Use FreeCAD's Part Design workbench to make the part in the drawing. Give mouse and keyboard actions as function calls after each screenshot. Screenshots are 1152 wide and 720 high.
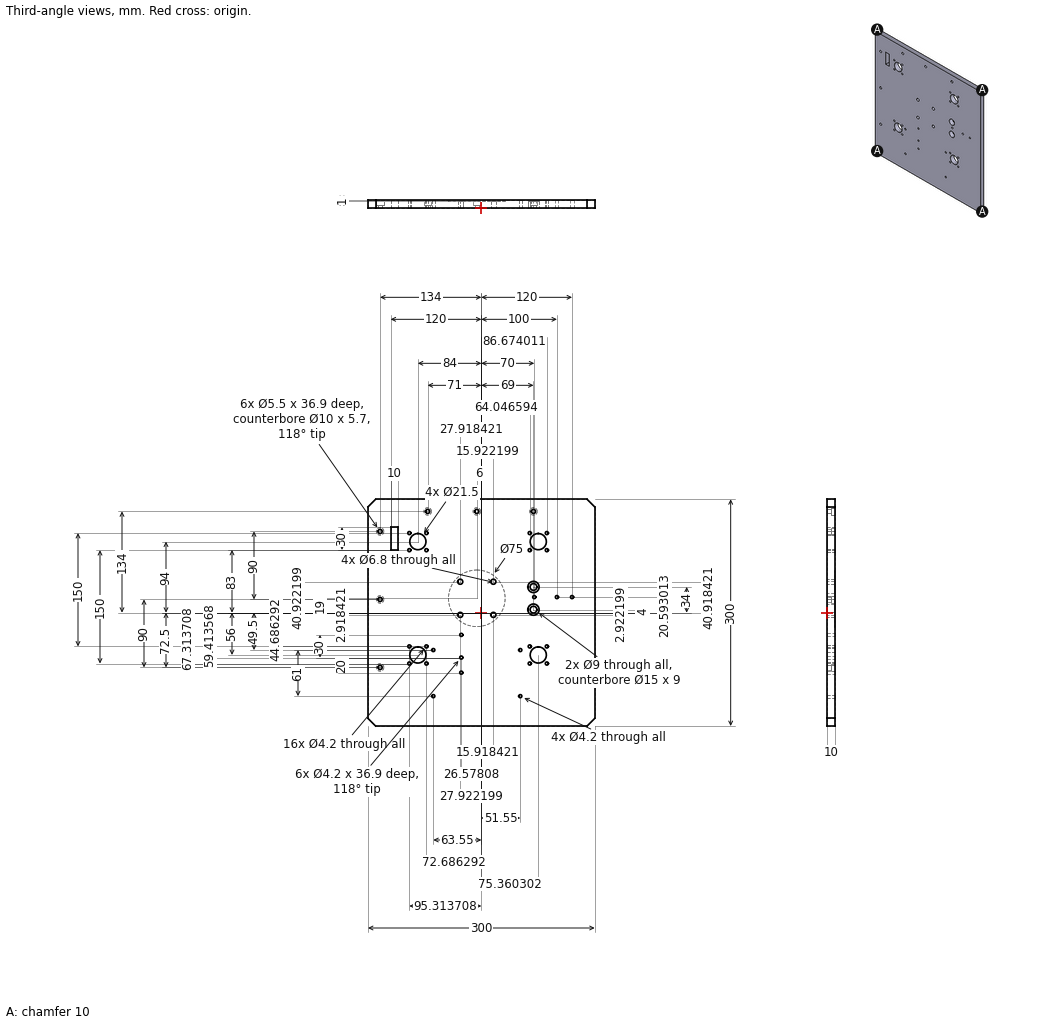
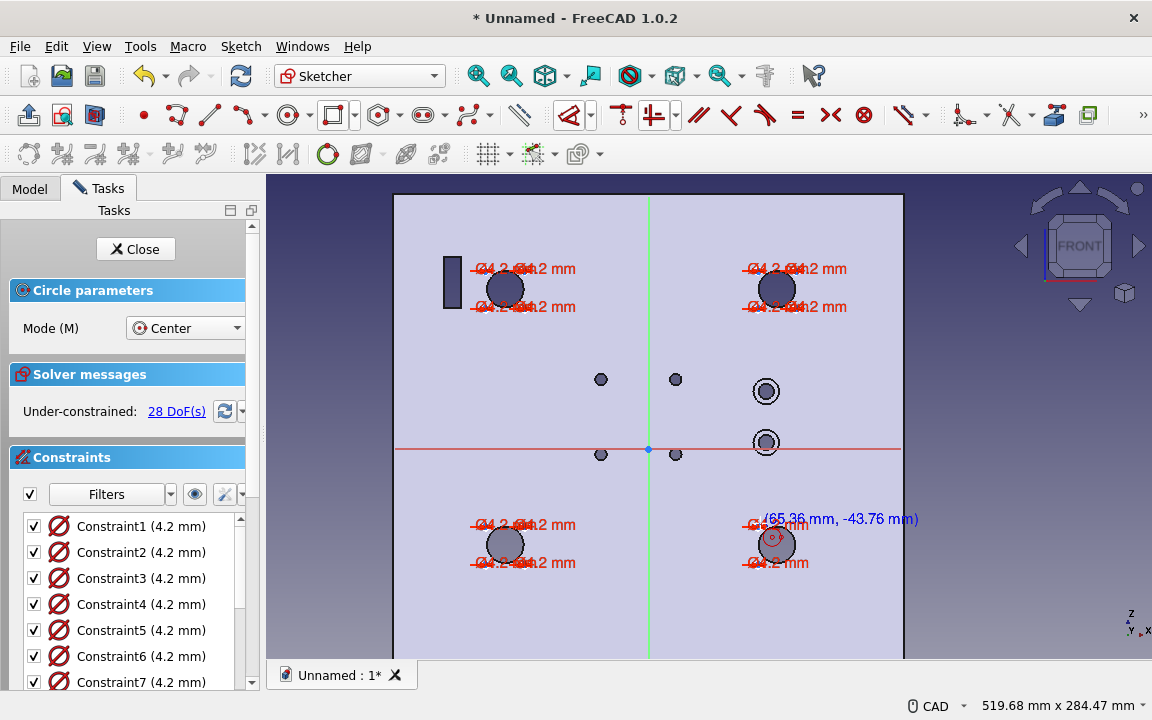
scroll(796, 526, up, 10)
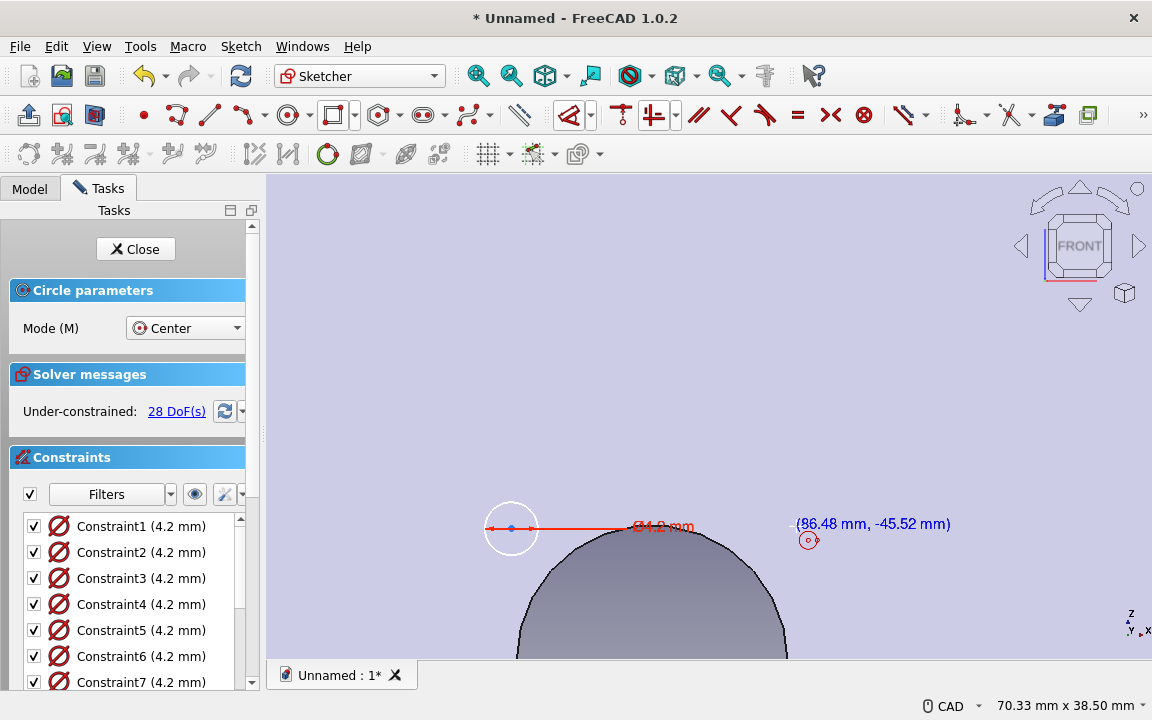
scroll(796, 526, down, 10)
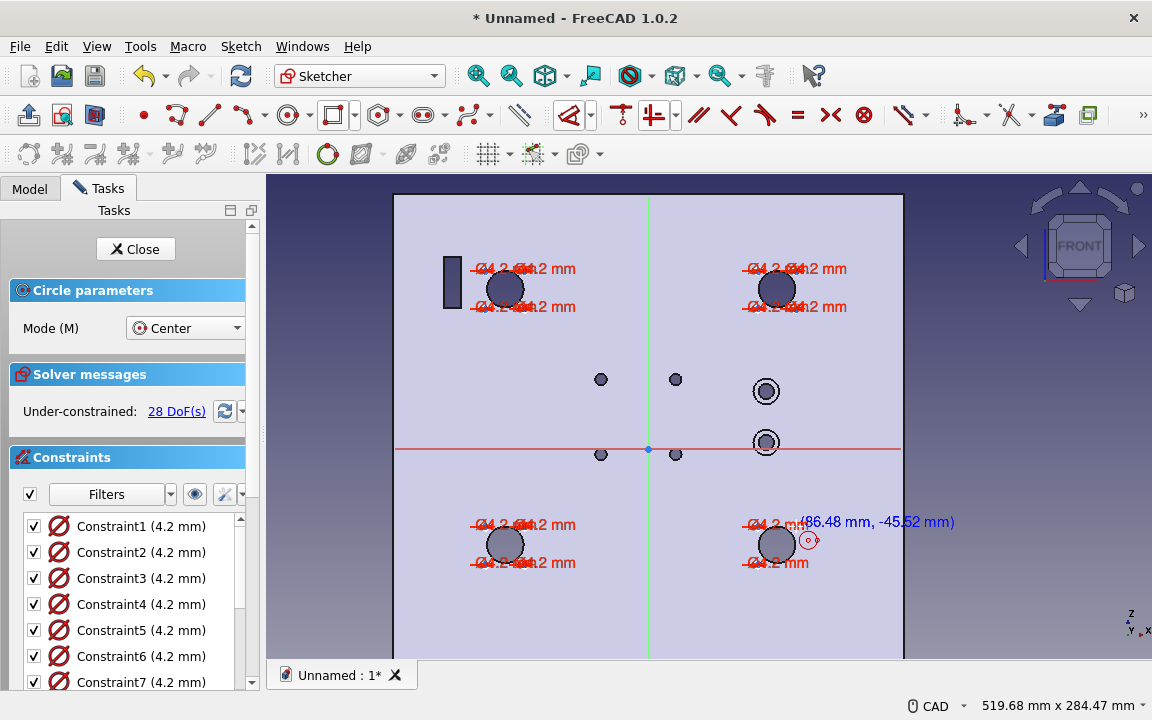
click(796, 526)
move(799, 523)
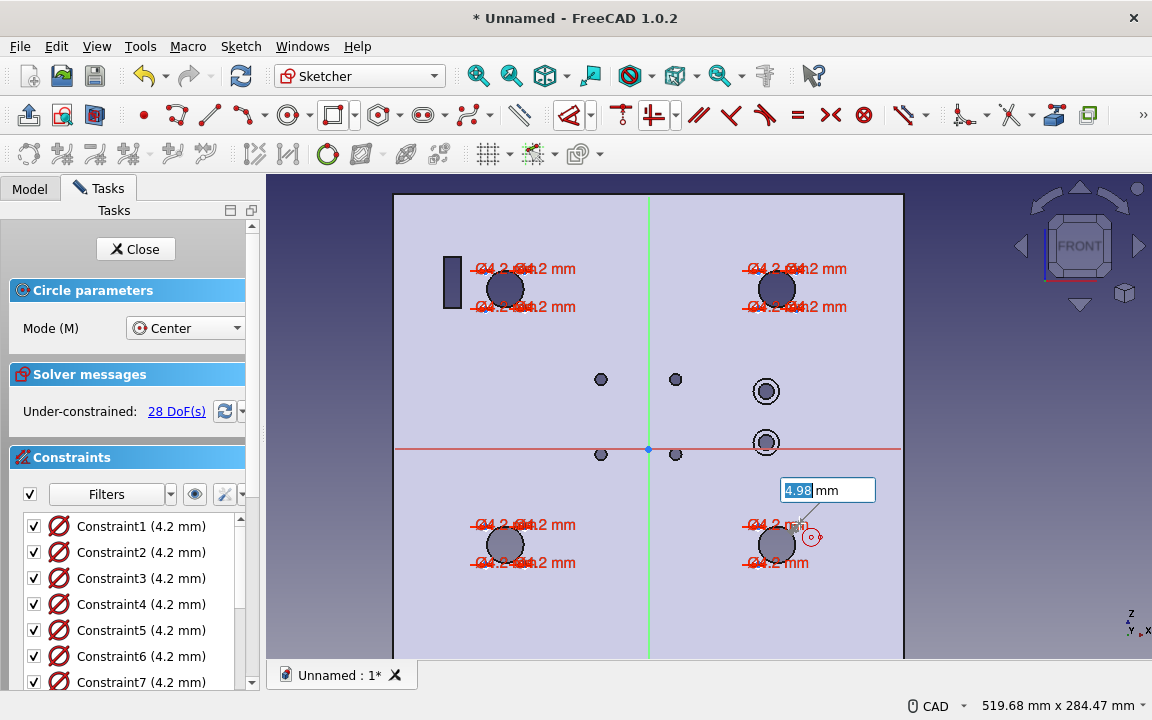
text(4.2)
key(Return)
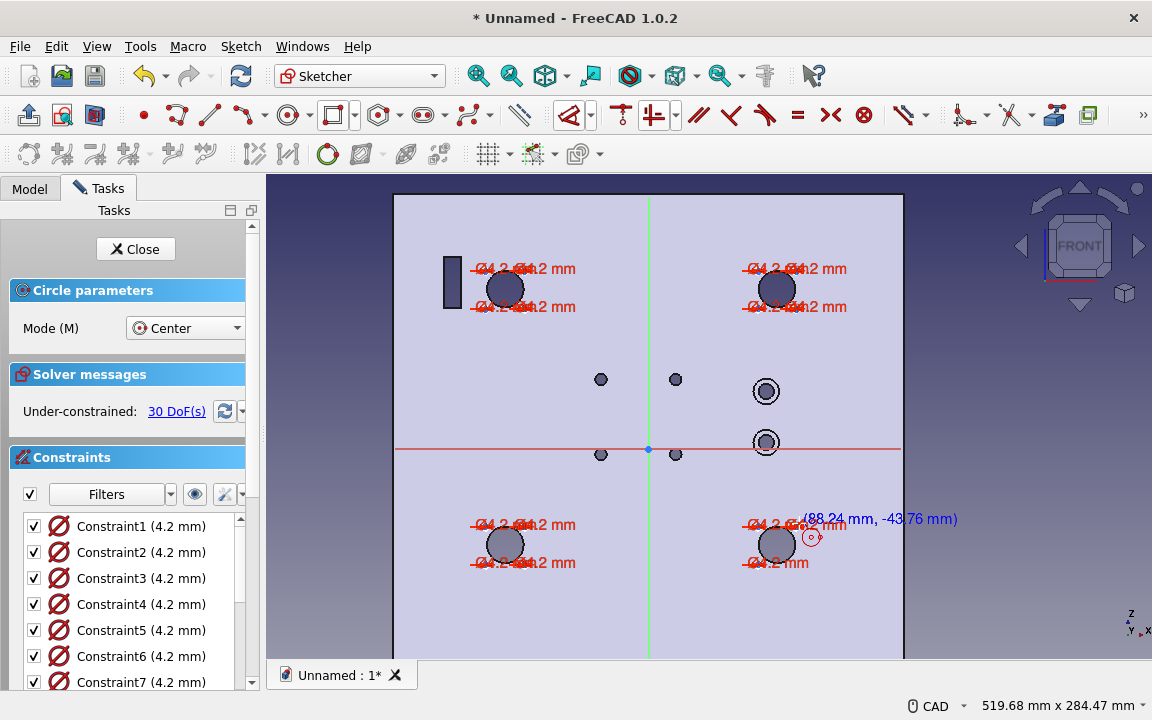
scroll(796, 564, up, 10)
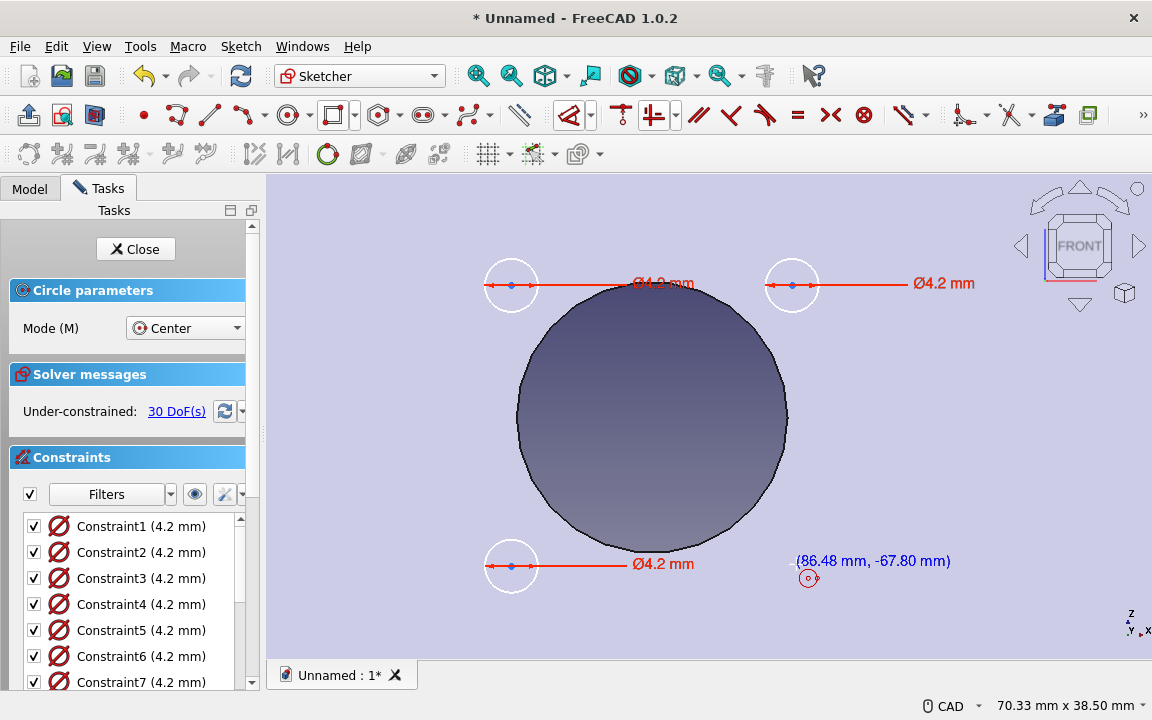
scroll(796, 564, down, 10)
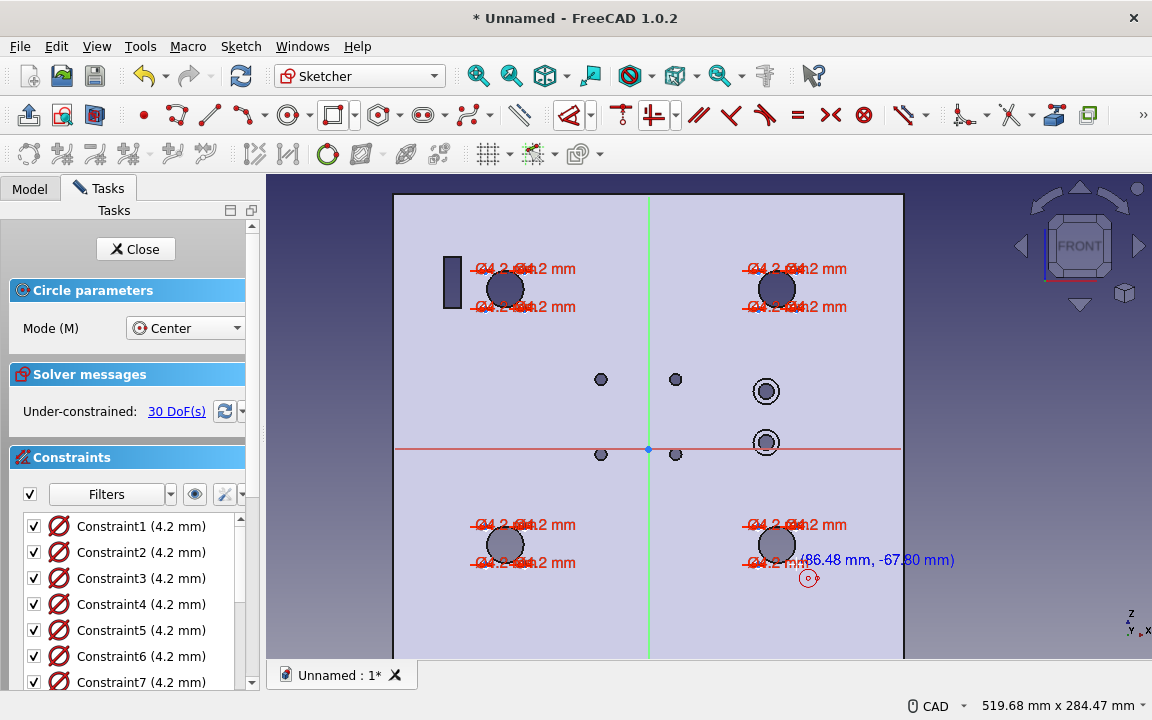
click(796, 564)
move(799, 562)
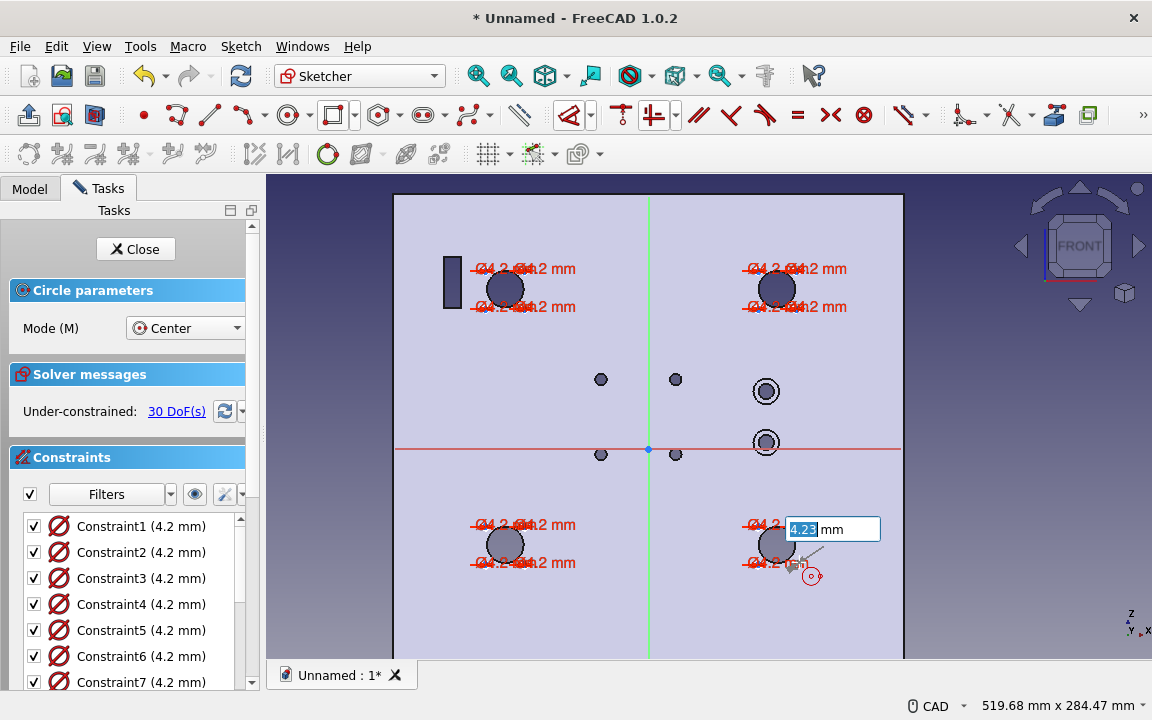
text(4.2)
key(Return)
key(Escape)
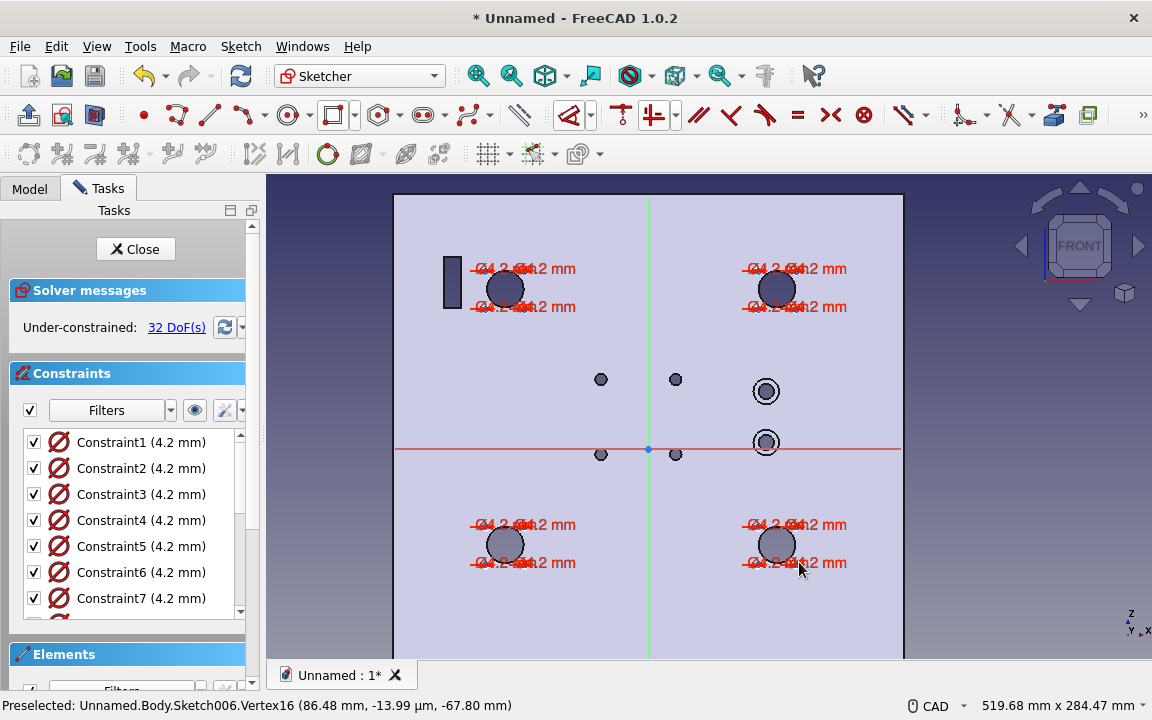
click(525, 527)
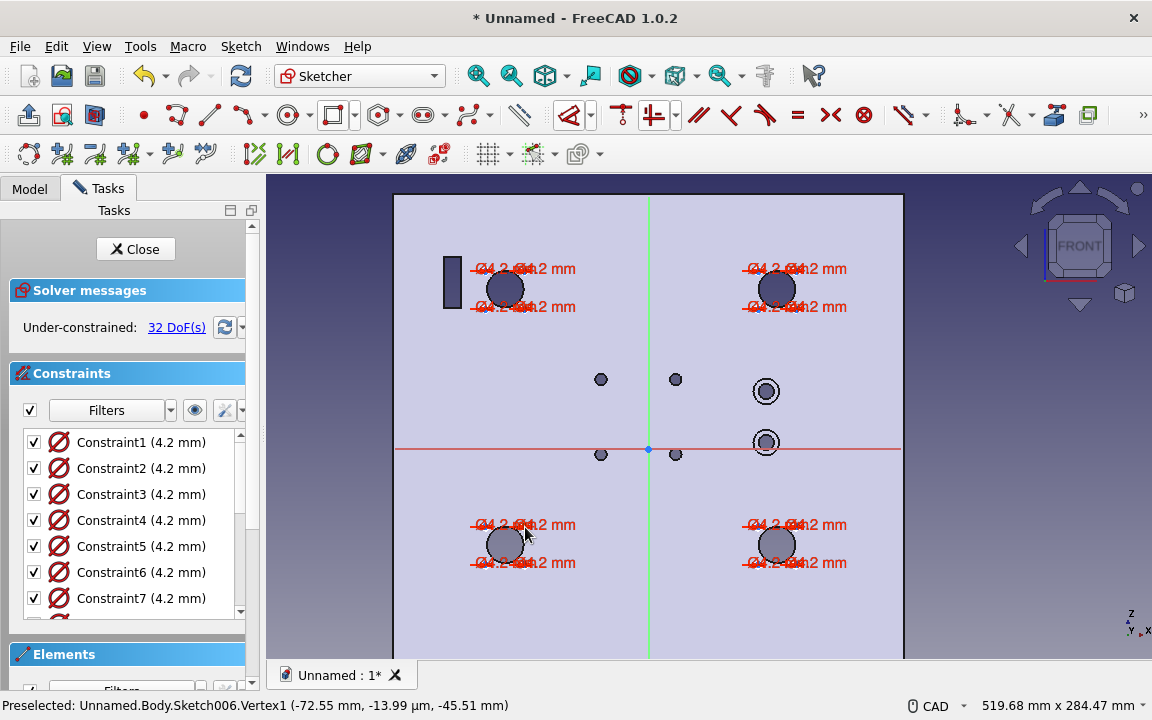
click(486, 527)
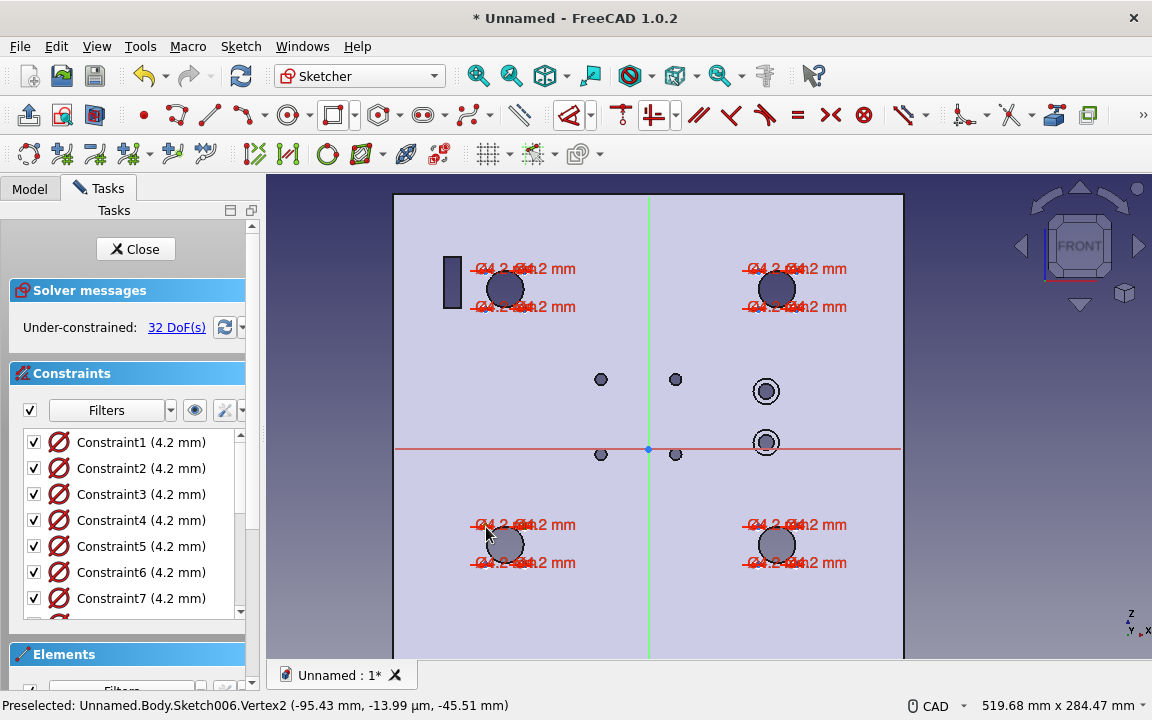
key(h)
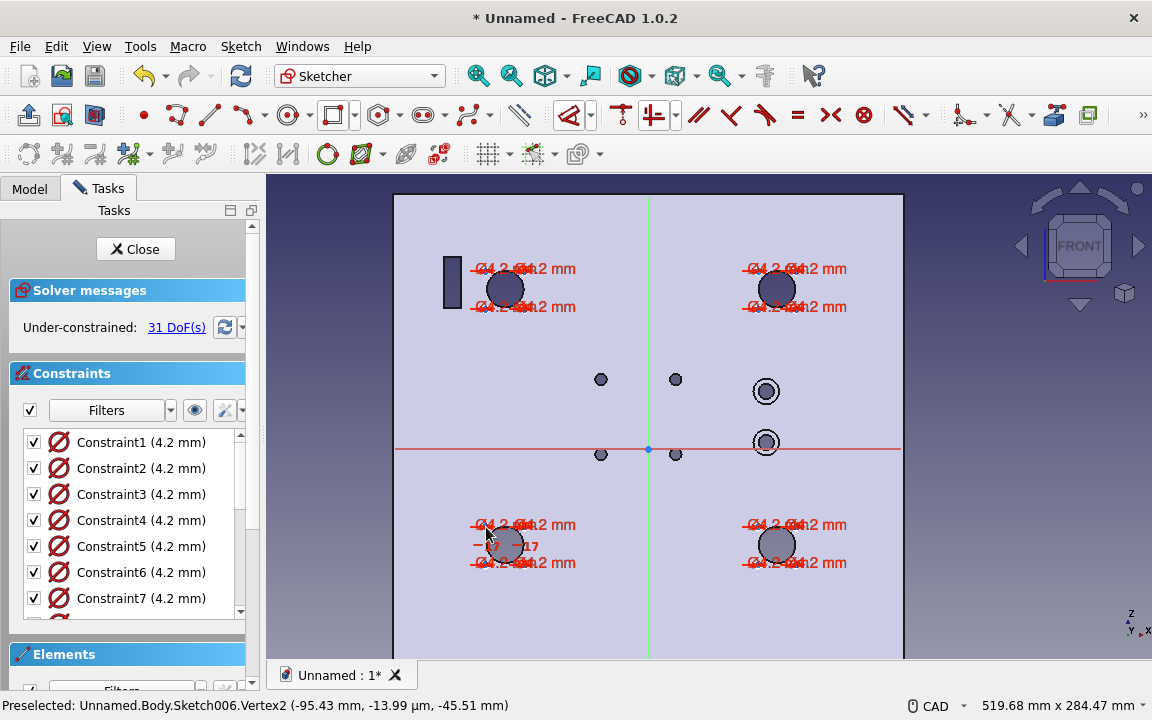
click(486, 527)